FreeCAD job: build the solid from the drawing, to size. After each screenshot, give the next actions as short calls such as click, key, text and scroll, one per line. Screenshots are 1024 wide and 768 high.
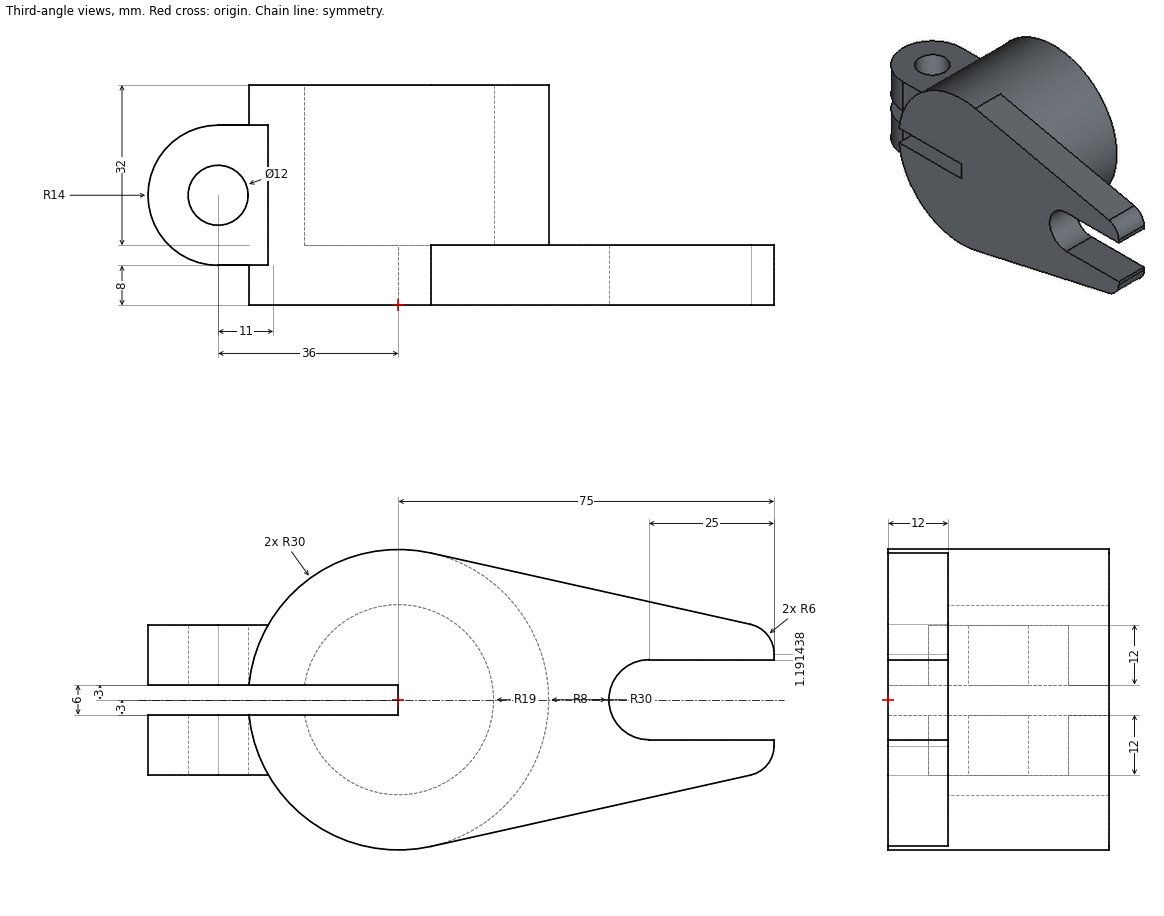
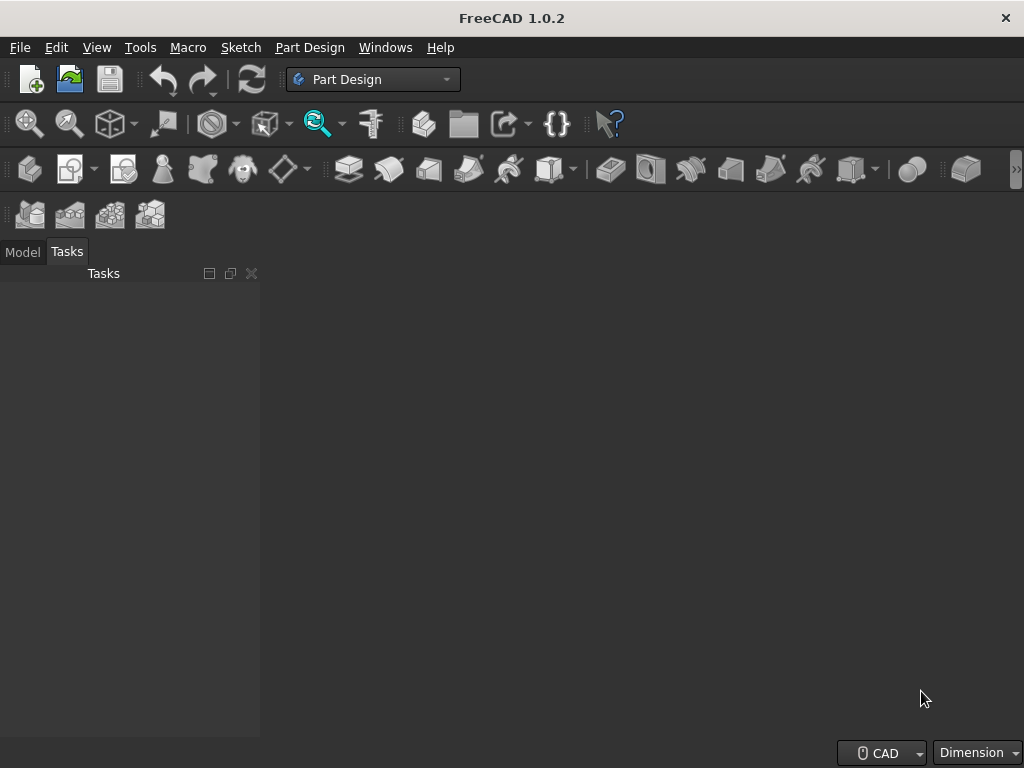
click(30, 80)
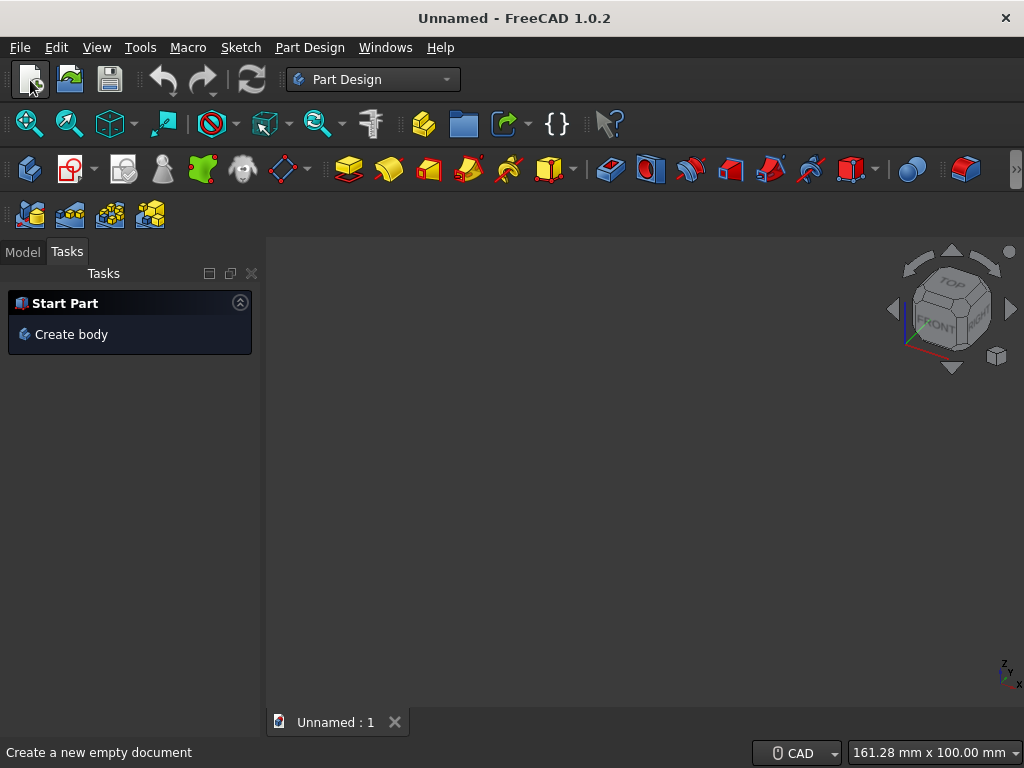
click(70, 170)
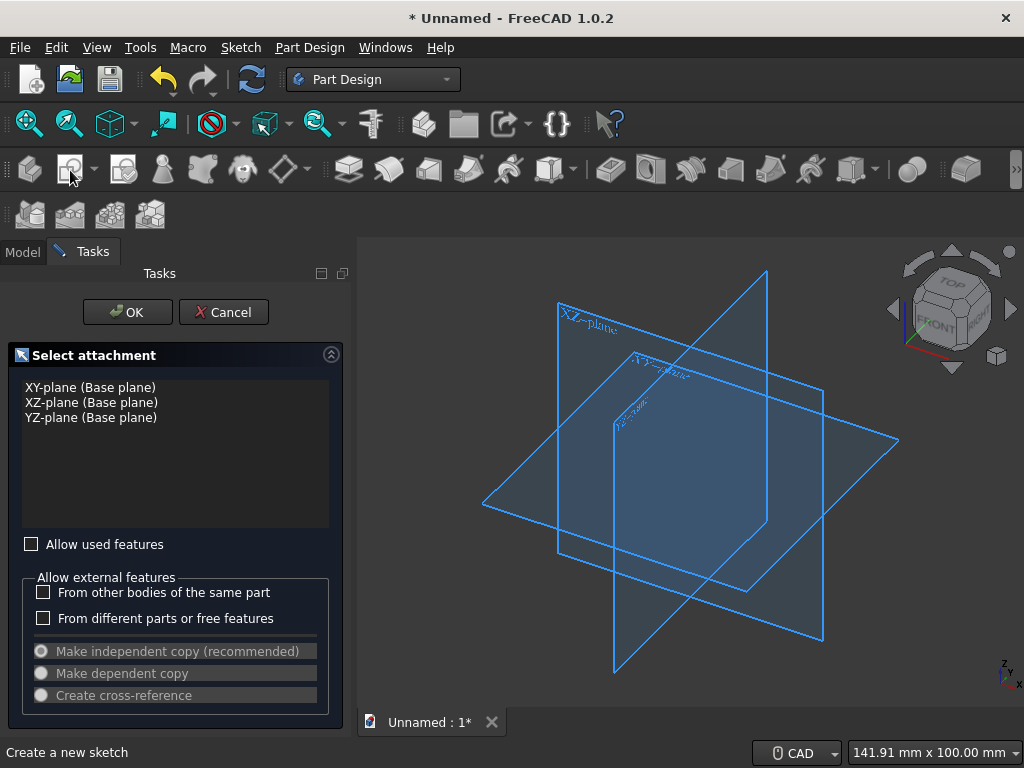
click(82, 402)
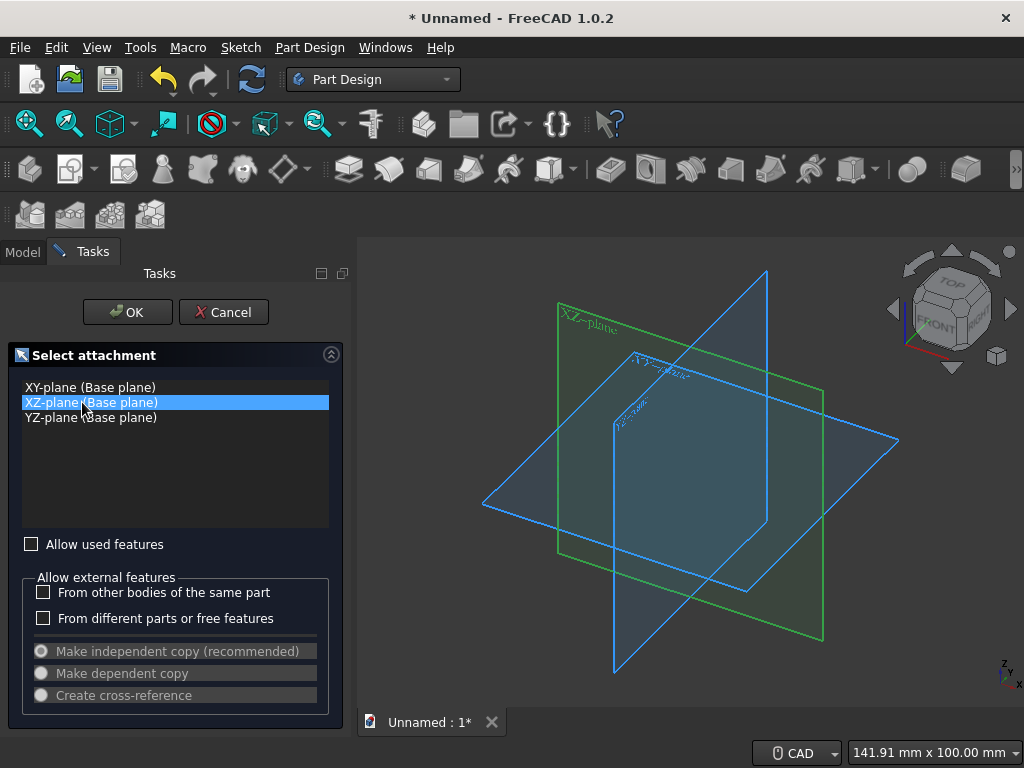
click(128, 312)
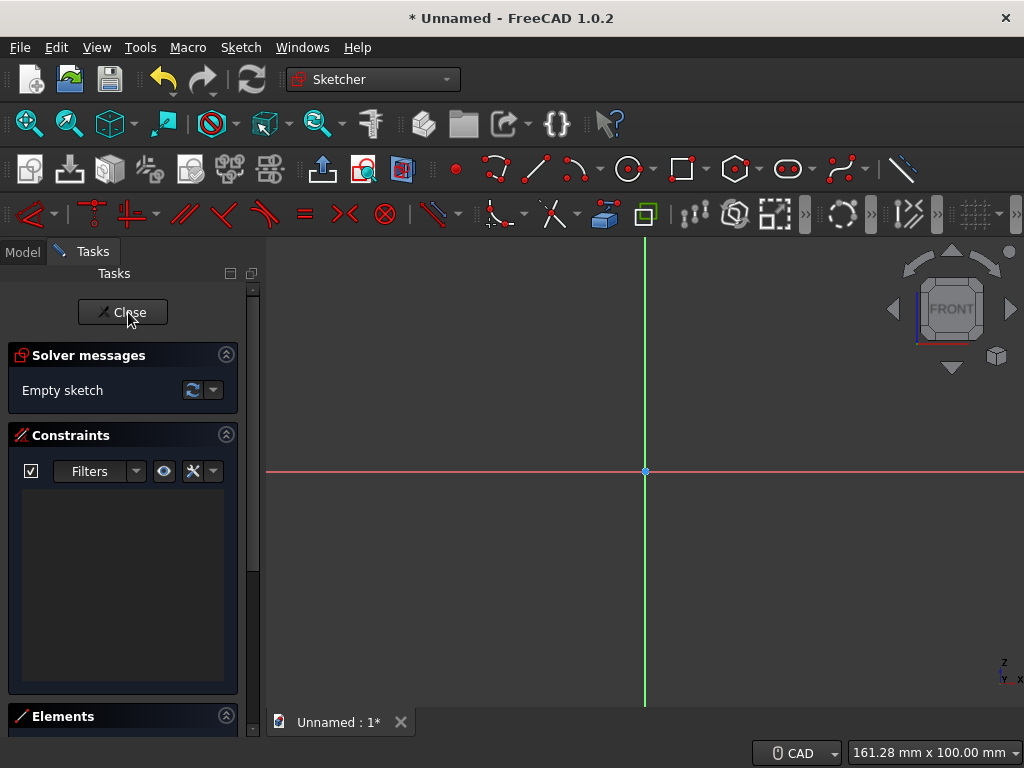
scroll(294, 472, down, 2)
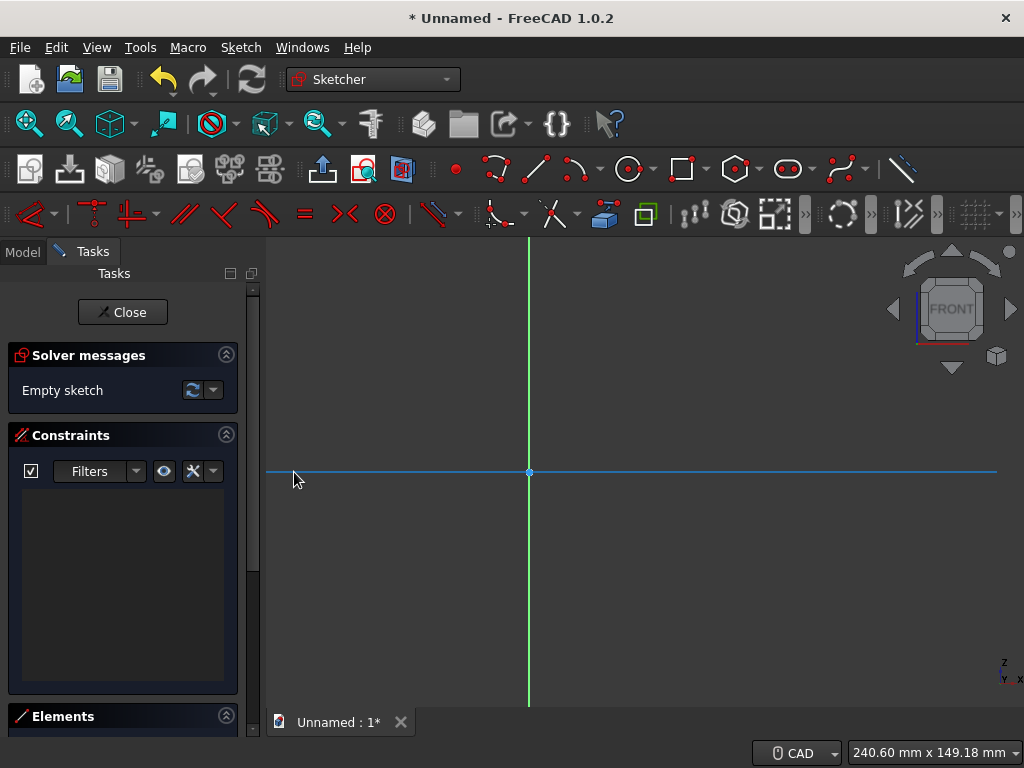
click(496, 170)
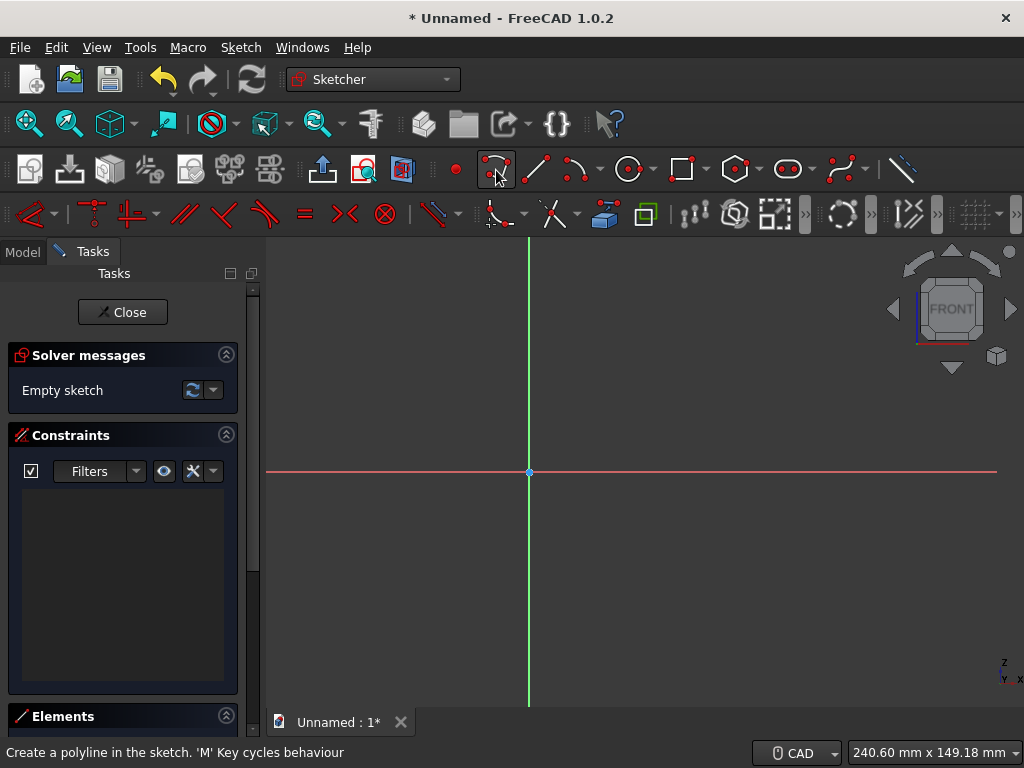
scroll(435, 482, up, 3)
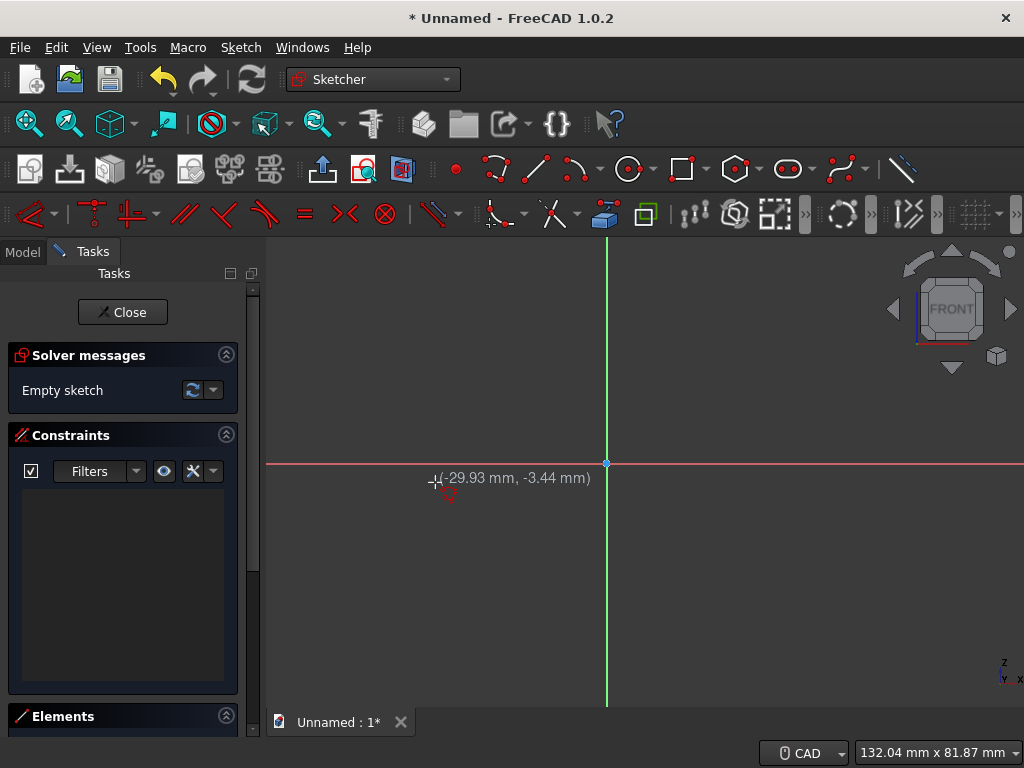
click(435, 481)
click(607, 481)
click(616, 446)
click(435, 446)
right_click(435, 446)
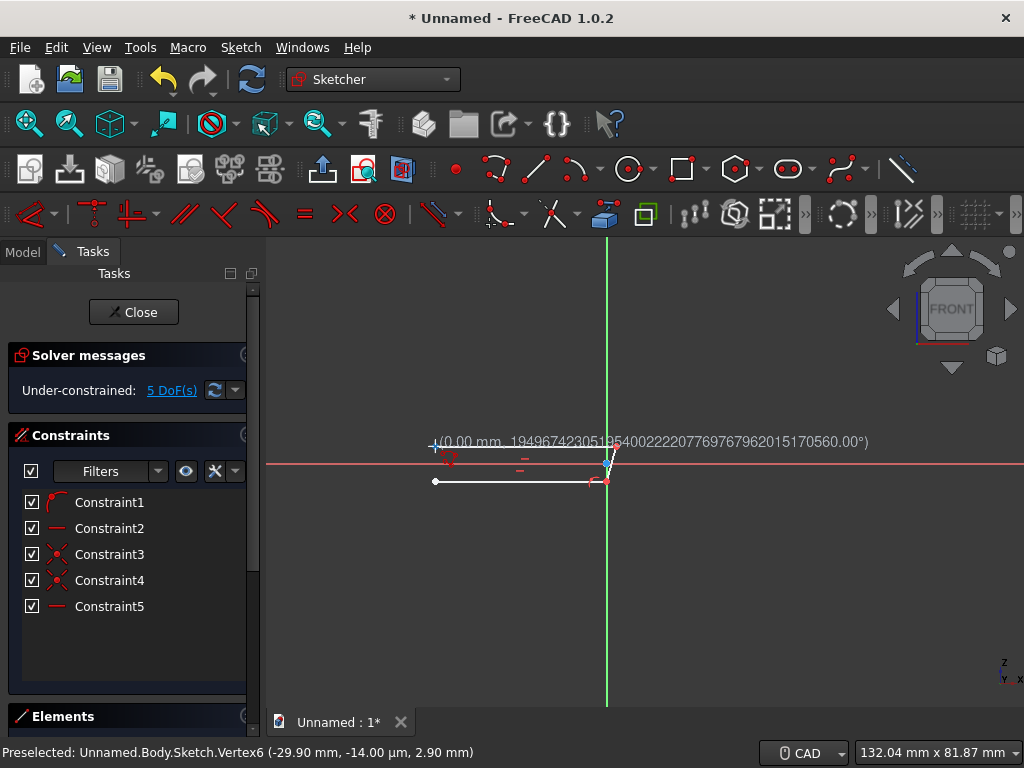
key(g)
key(l)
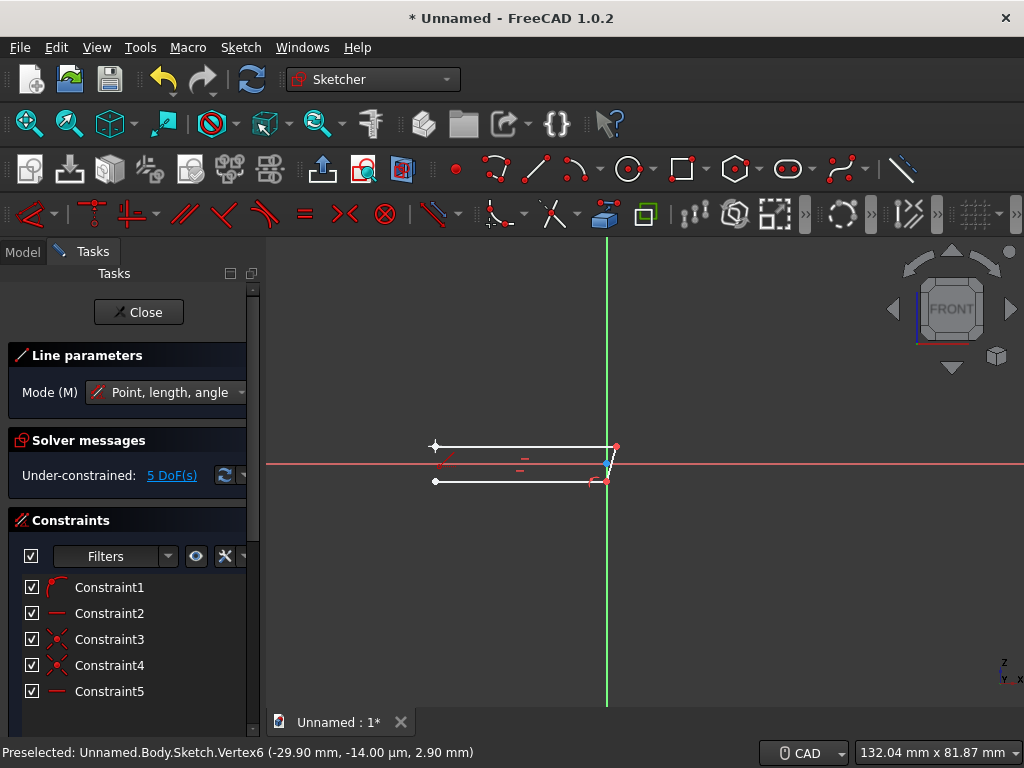
click(644, 296)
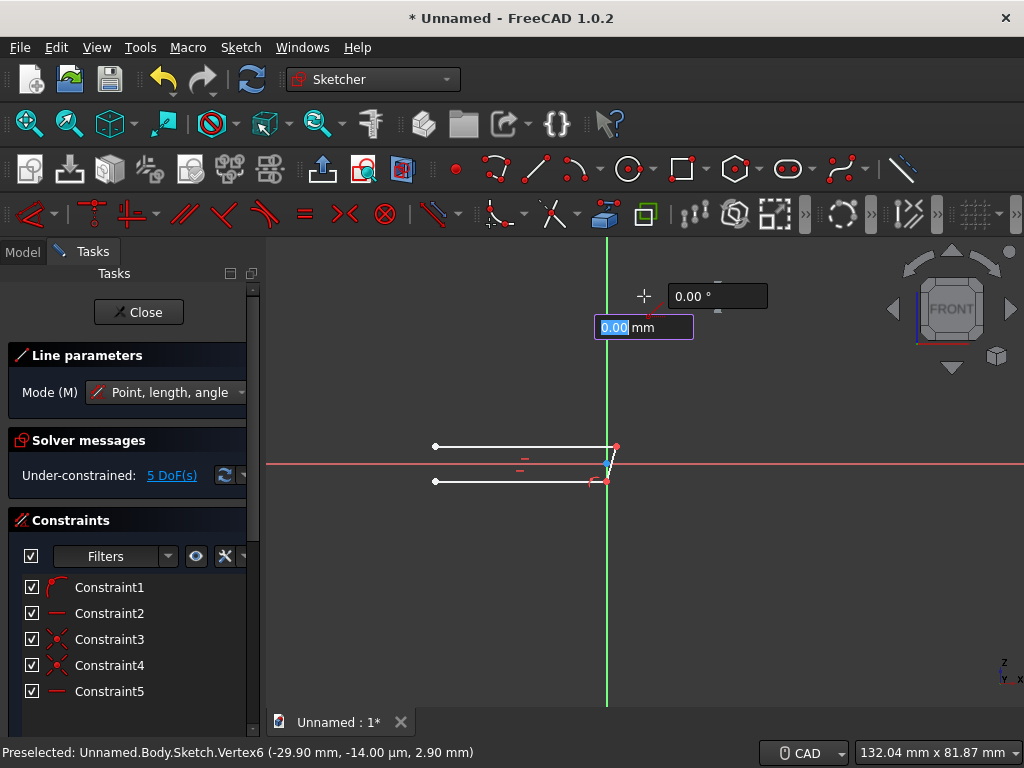
scroll(294, 489, down, 2)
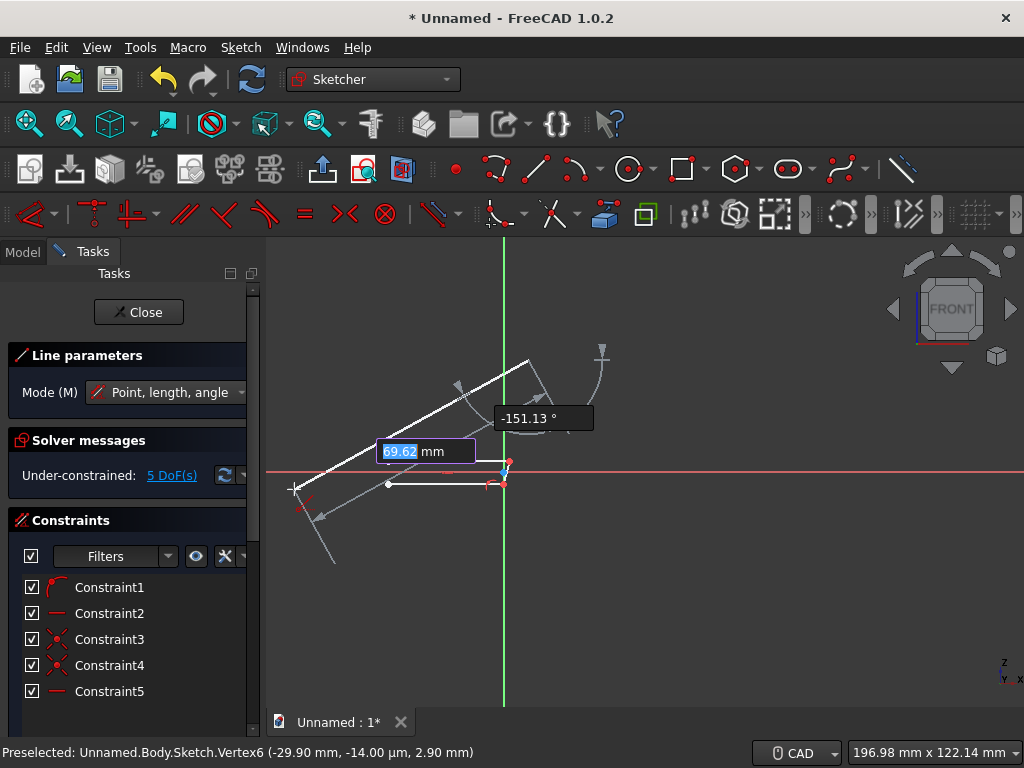
click(774, 414)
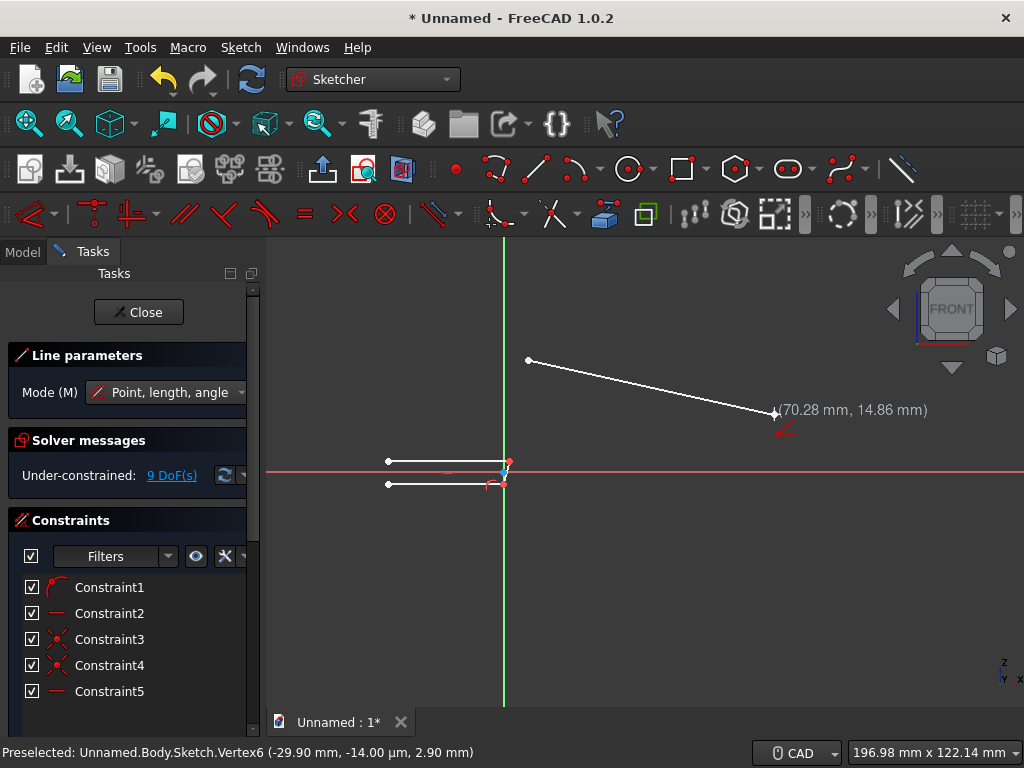
key(g)
key(m)